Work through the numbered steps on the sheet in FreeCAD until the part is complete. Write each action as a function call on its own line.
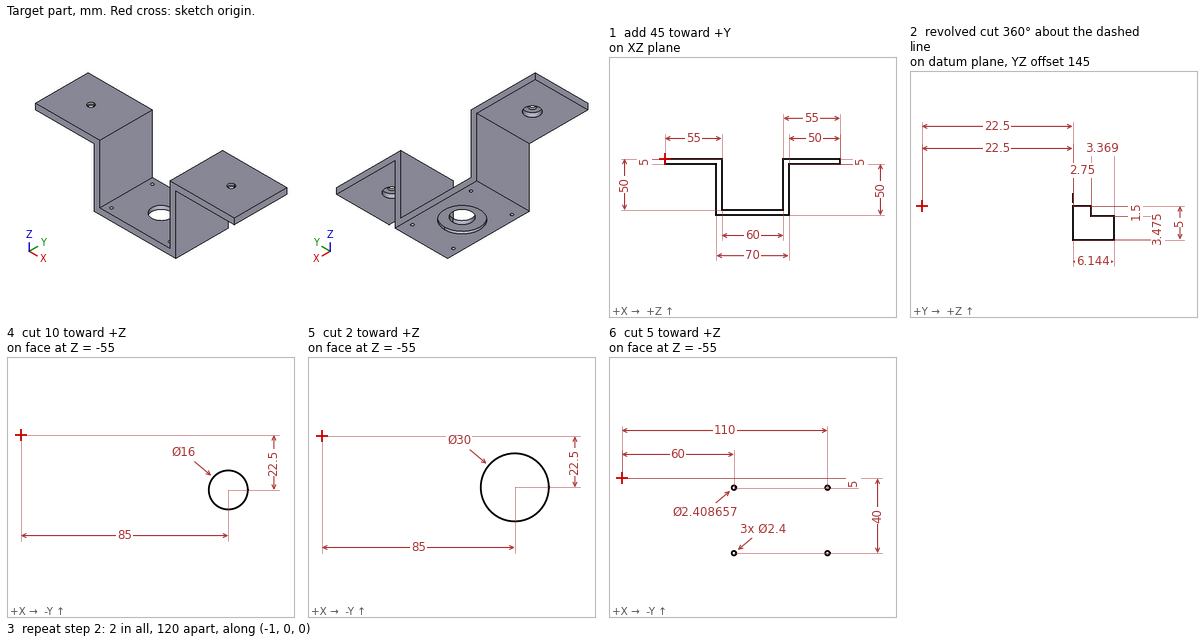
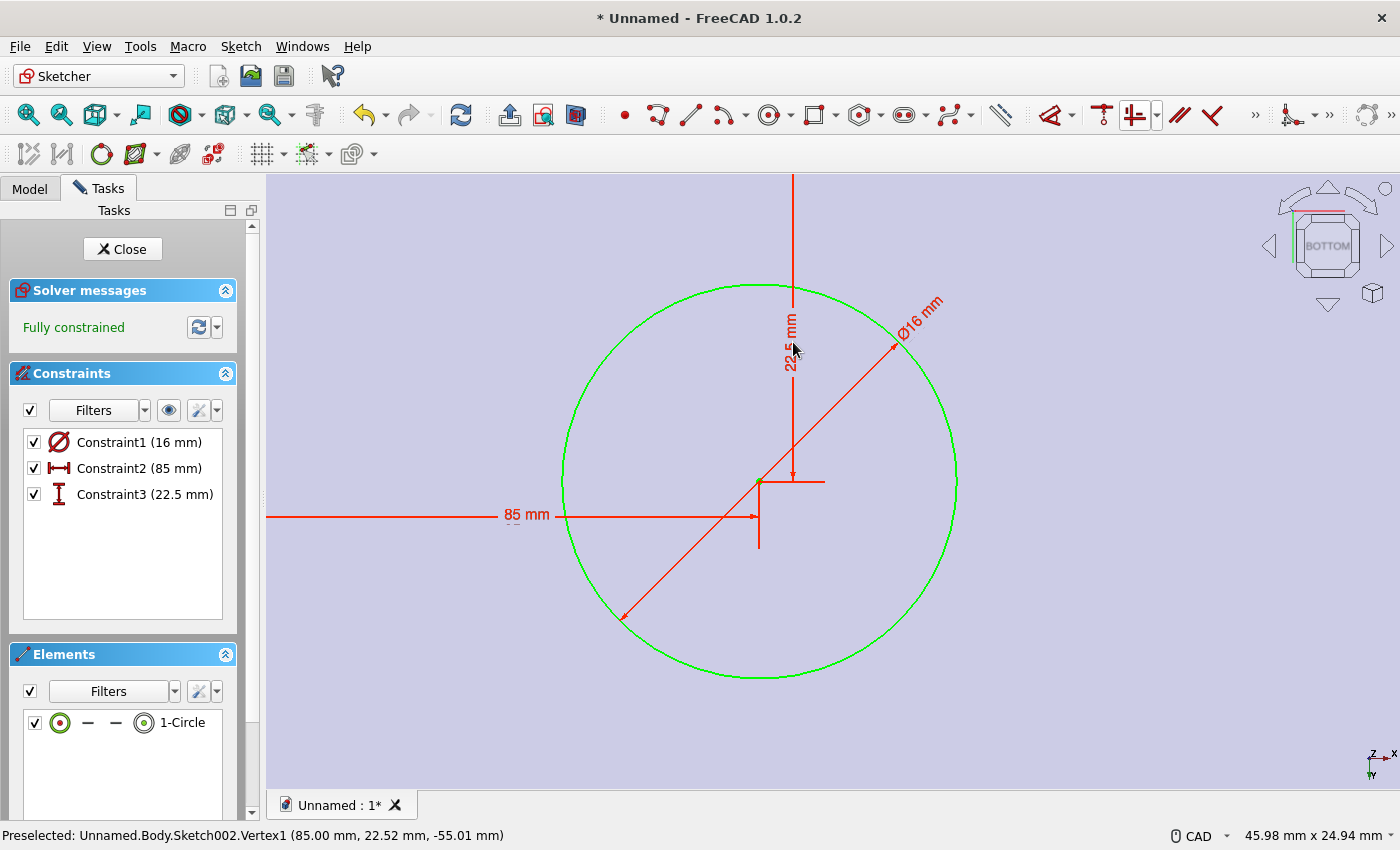
click(123, 249)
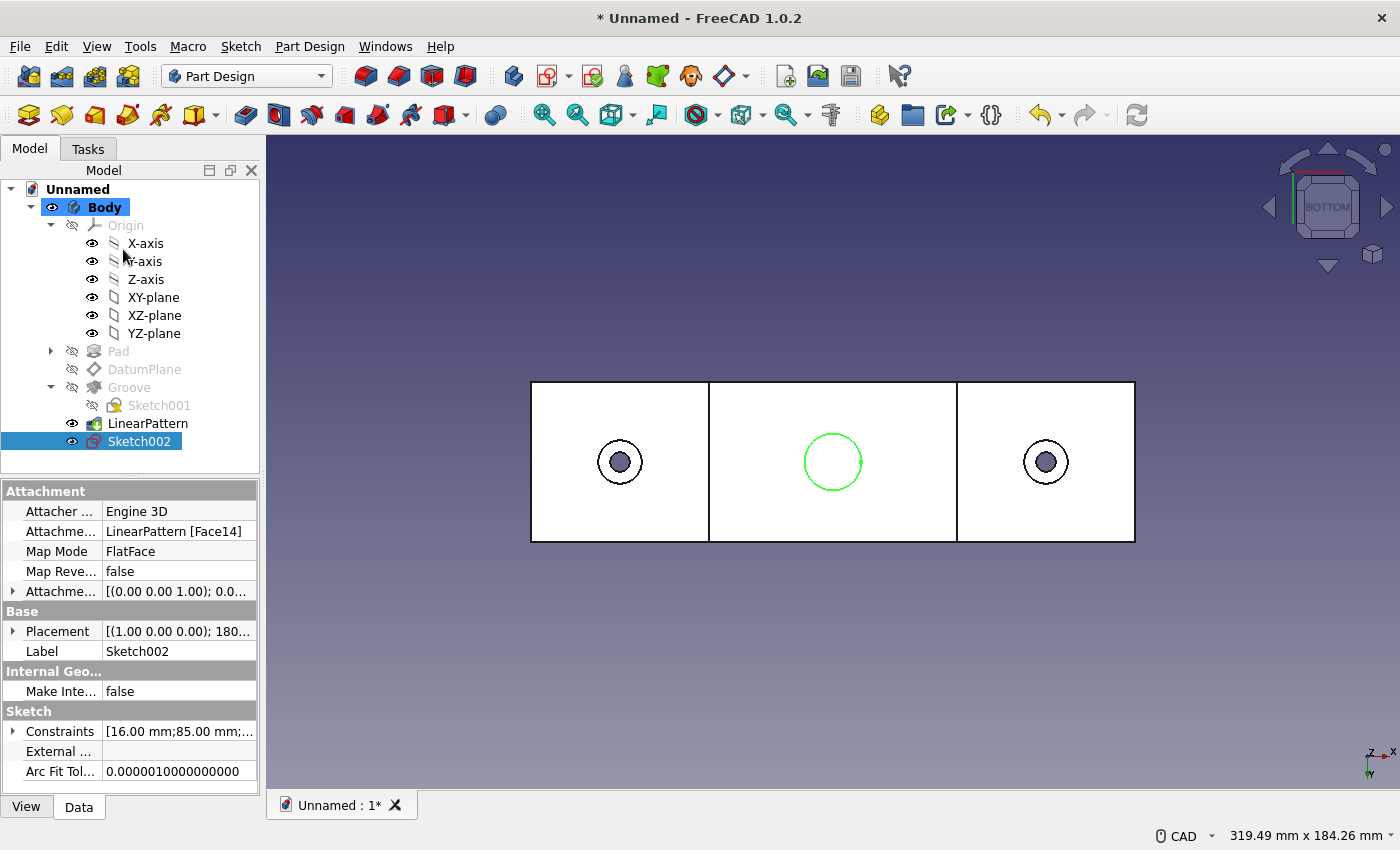
click(246, 116)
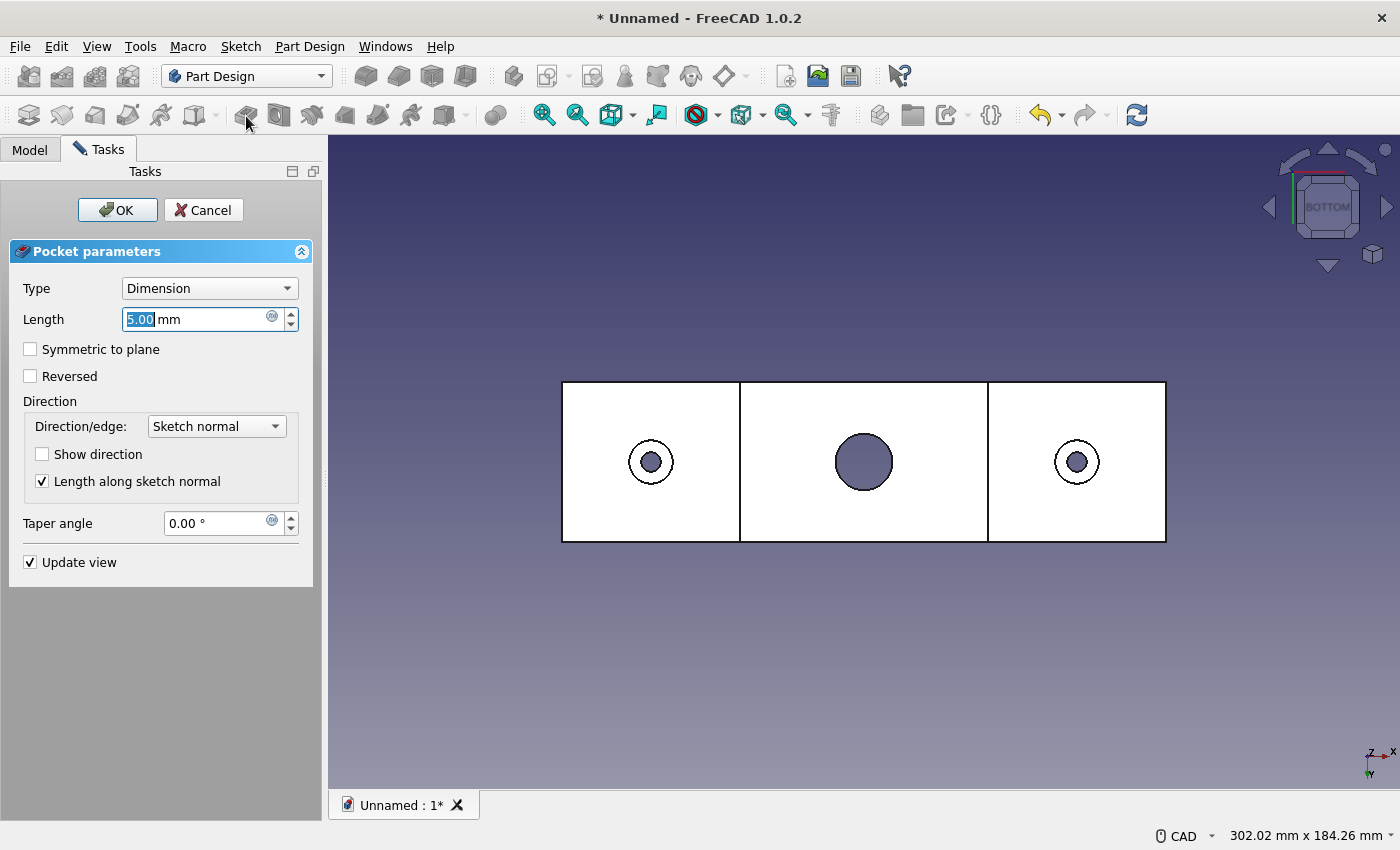
text(10)
key(Tab)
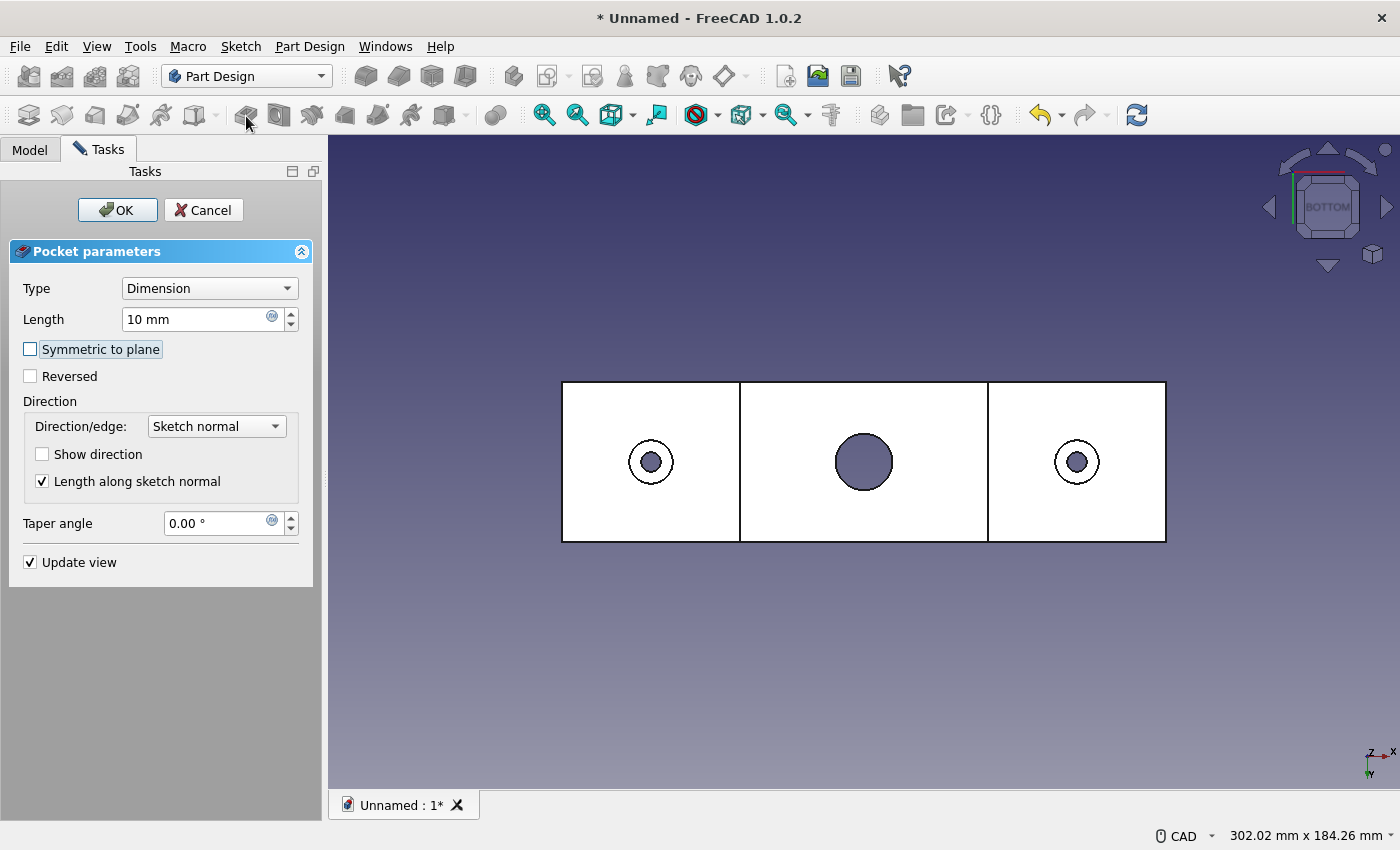
click(118, 210)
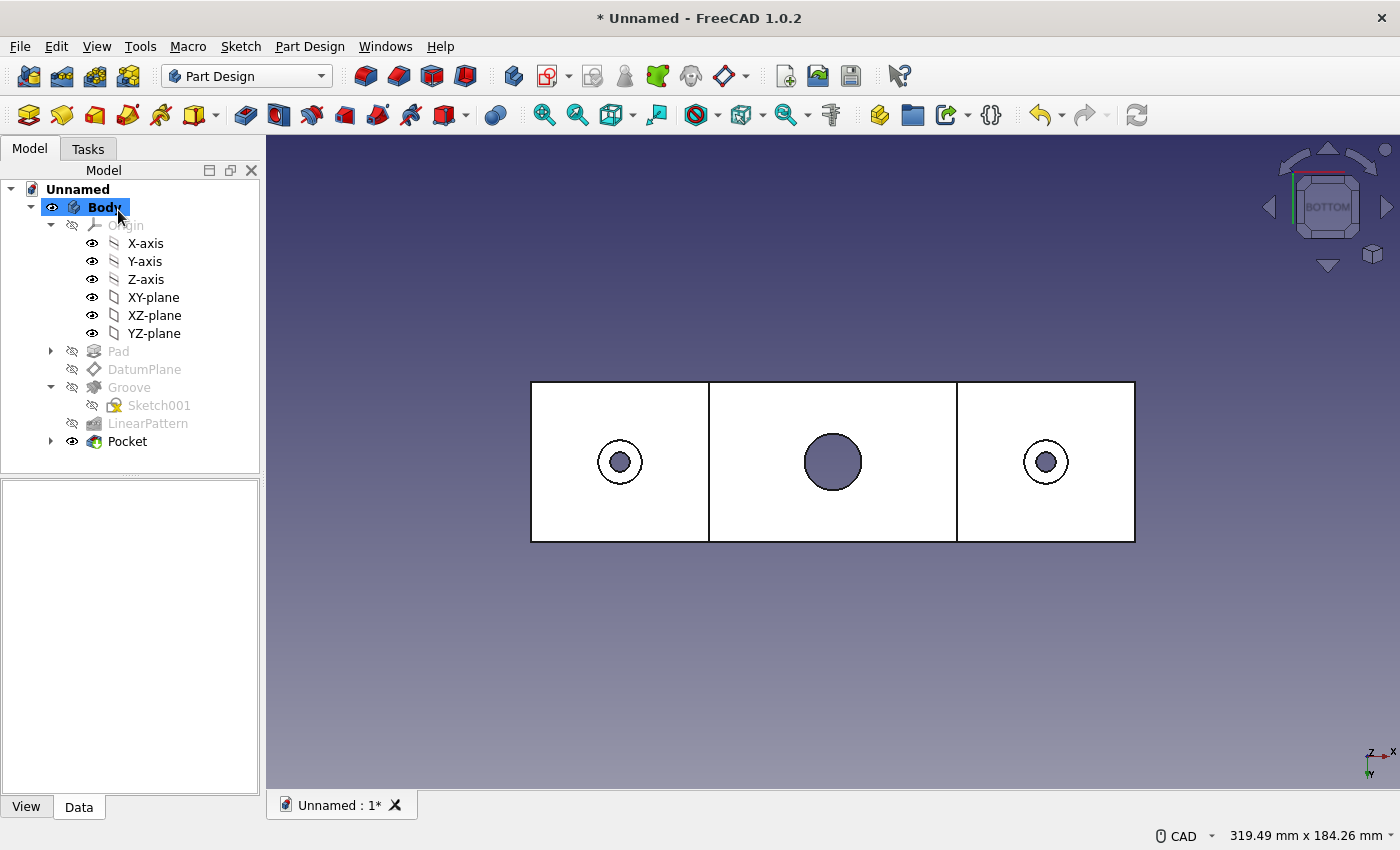
click(904, 484)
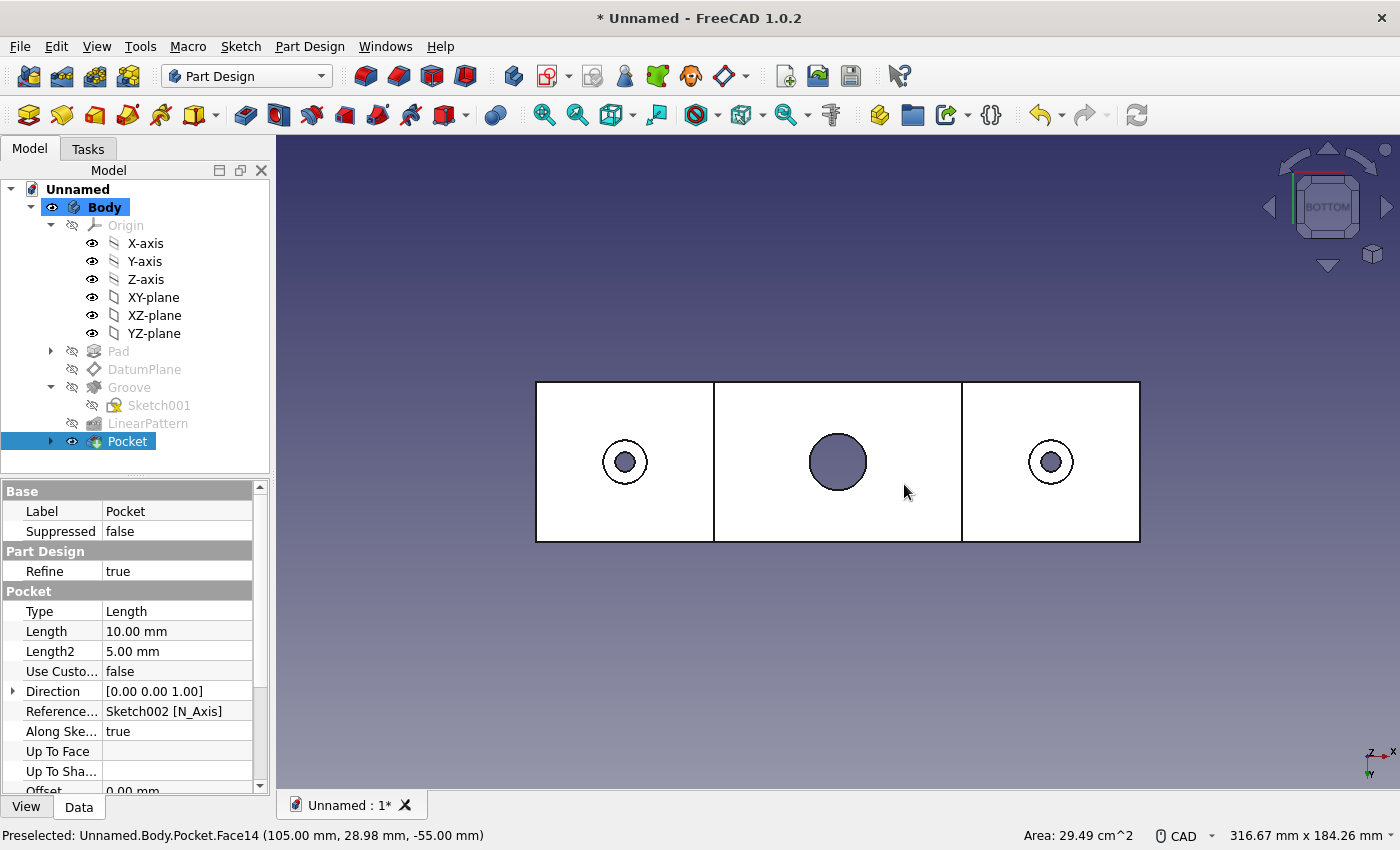
click(546, 76)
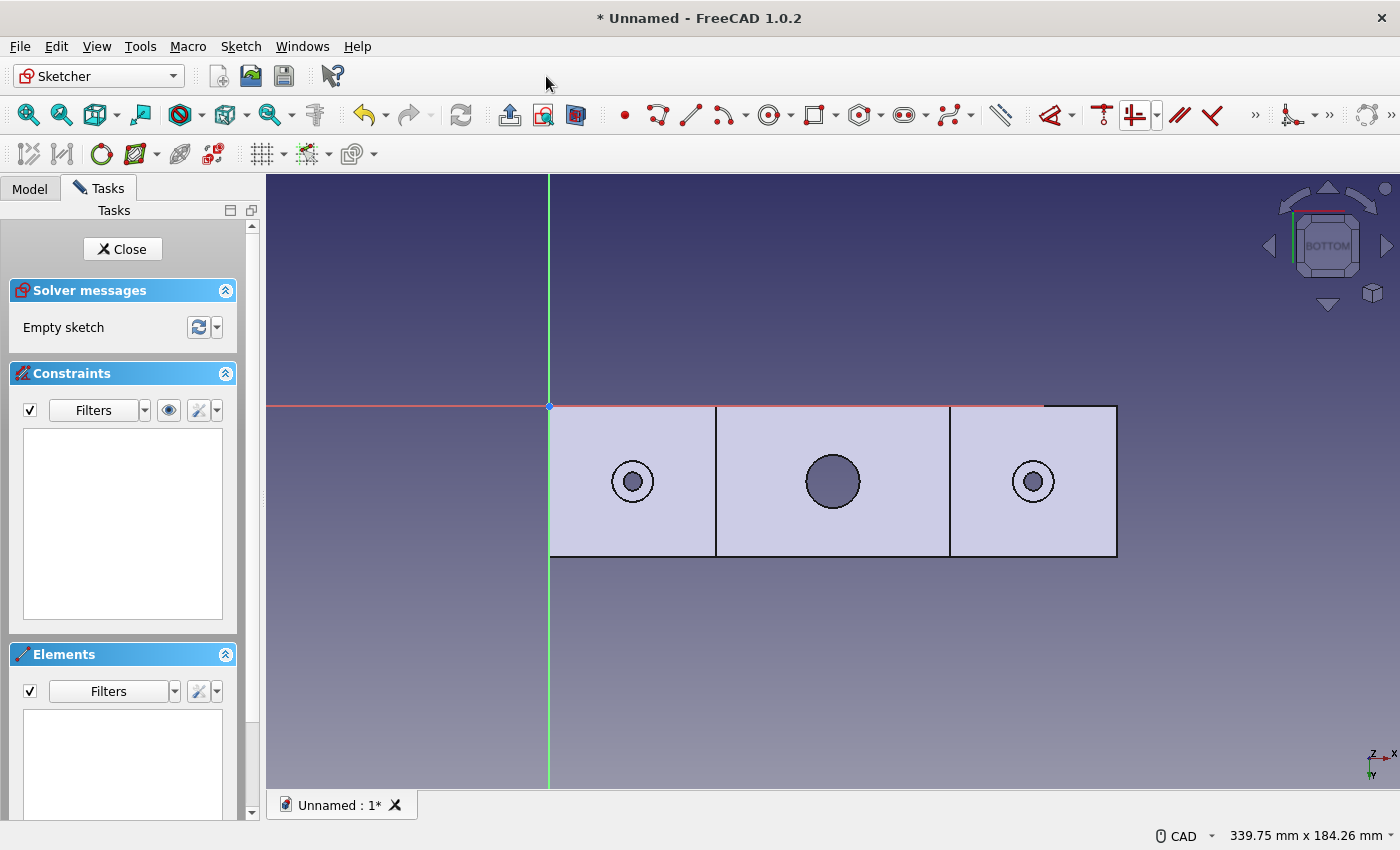
scroll(855, 481, up, 7)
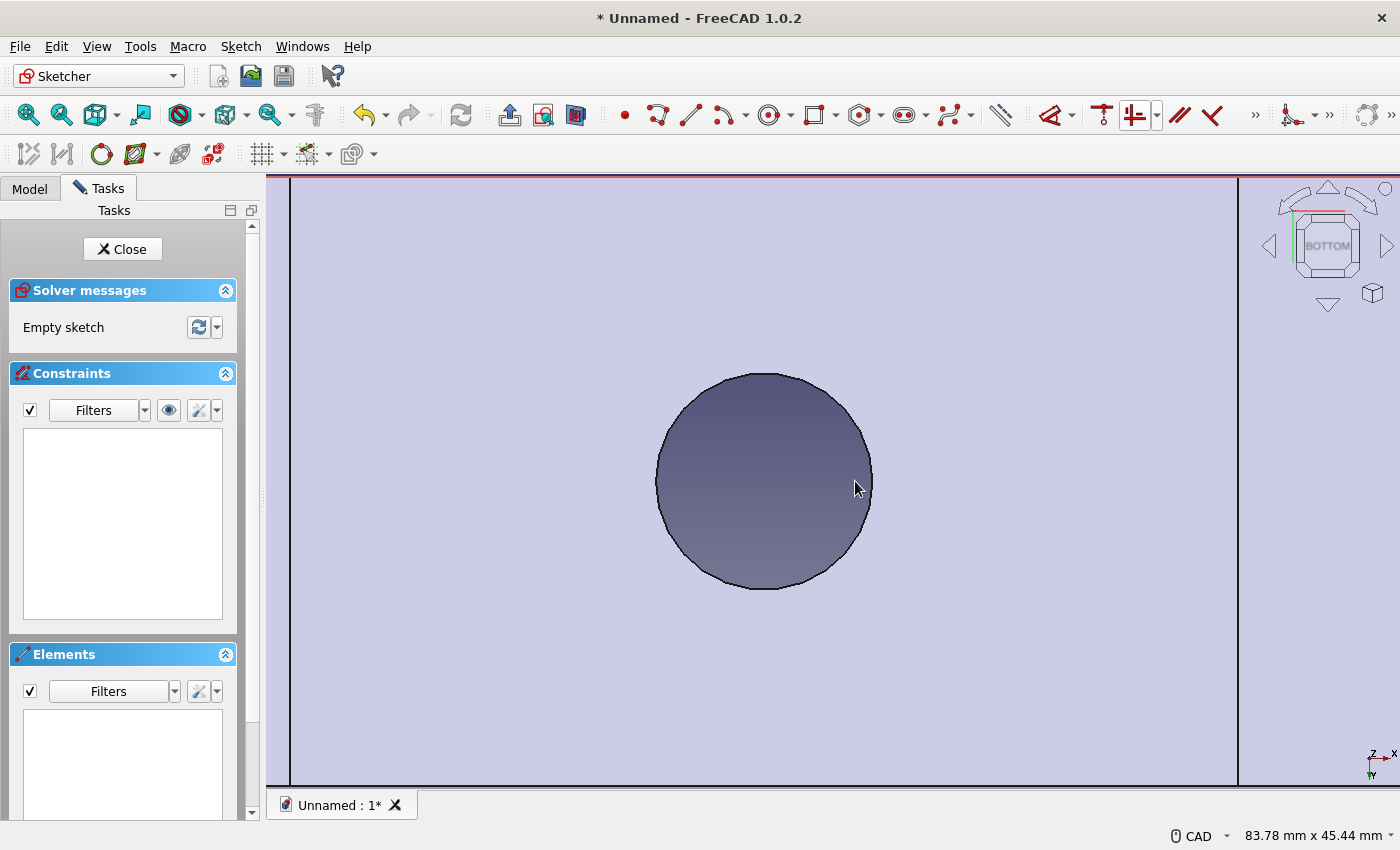
key(g)
key(c)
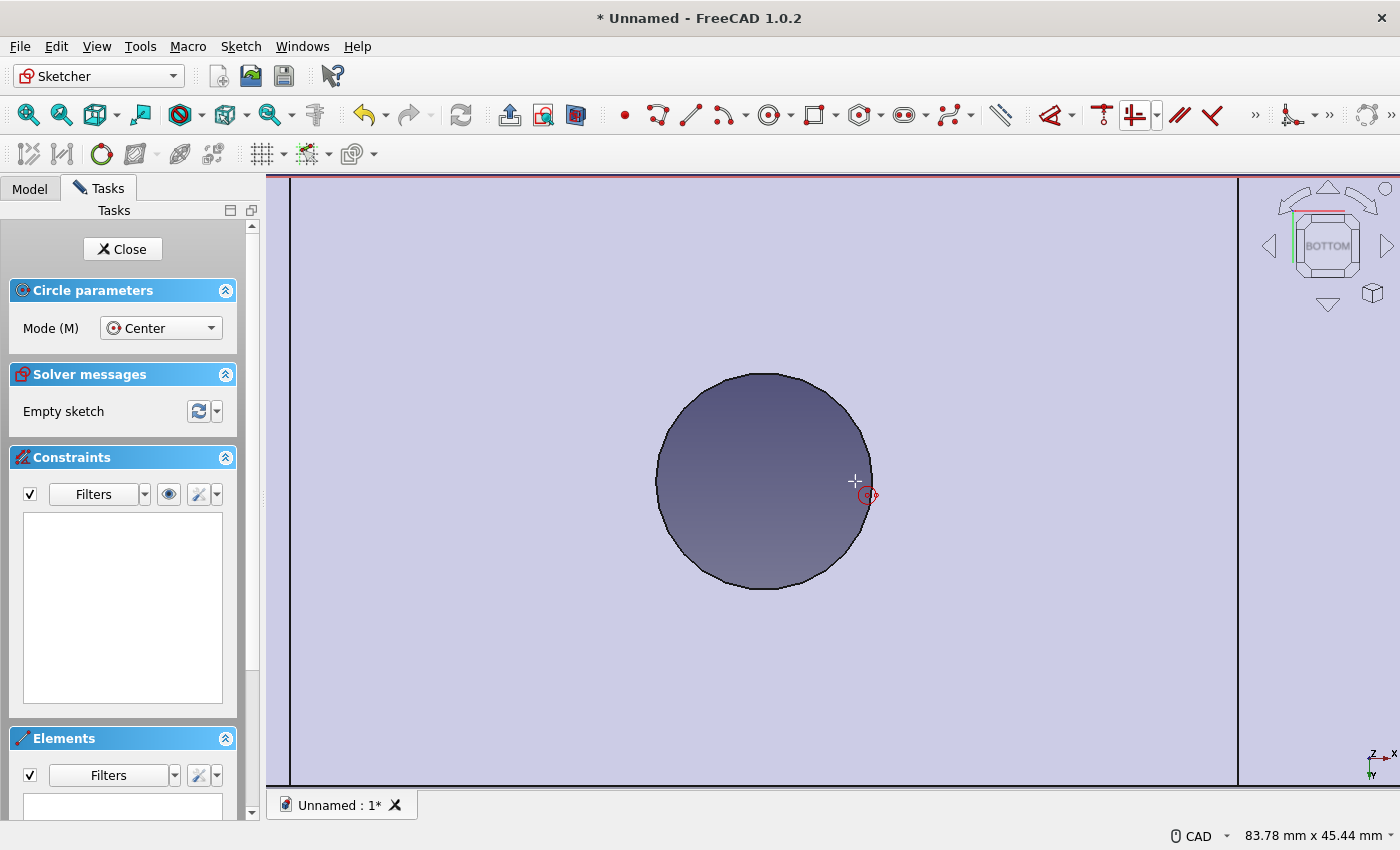
click(764, 481)
click(908, 338)
key(Escape)